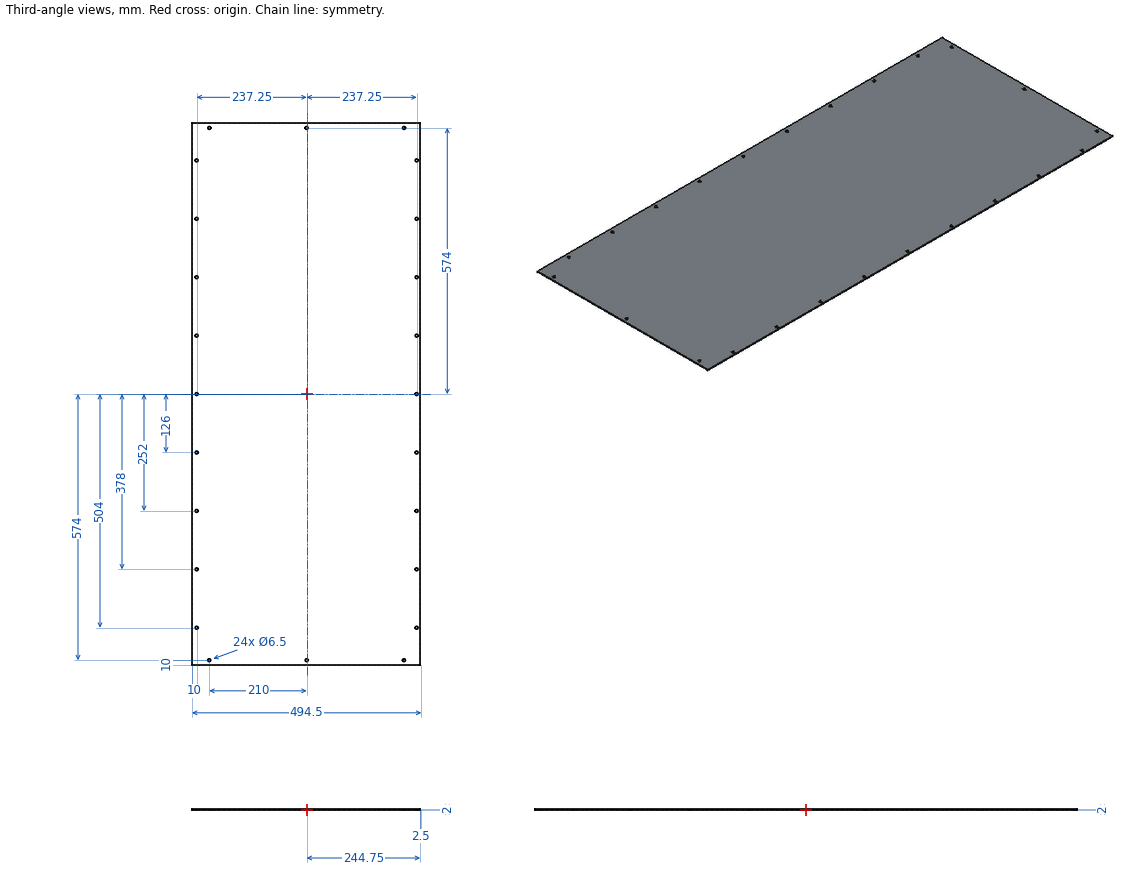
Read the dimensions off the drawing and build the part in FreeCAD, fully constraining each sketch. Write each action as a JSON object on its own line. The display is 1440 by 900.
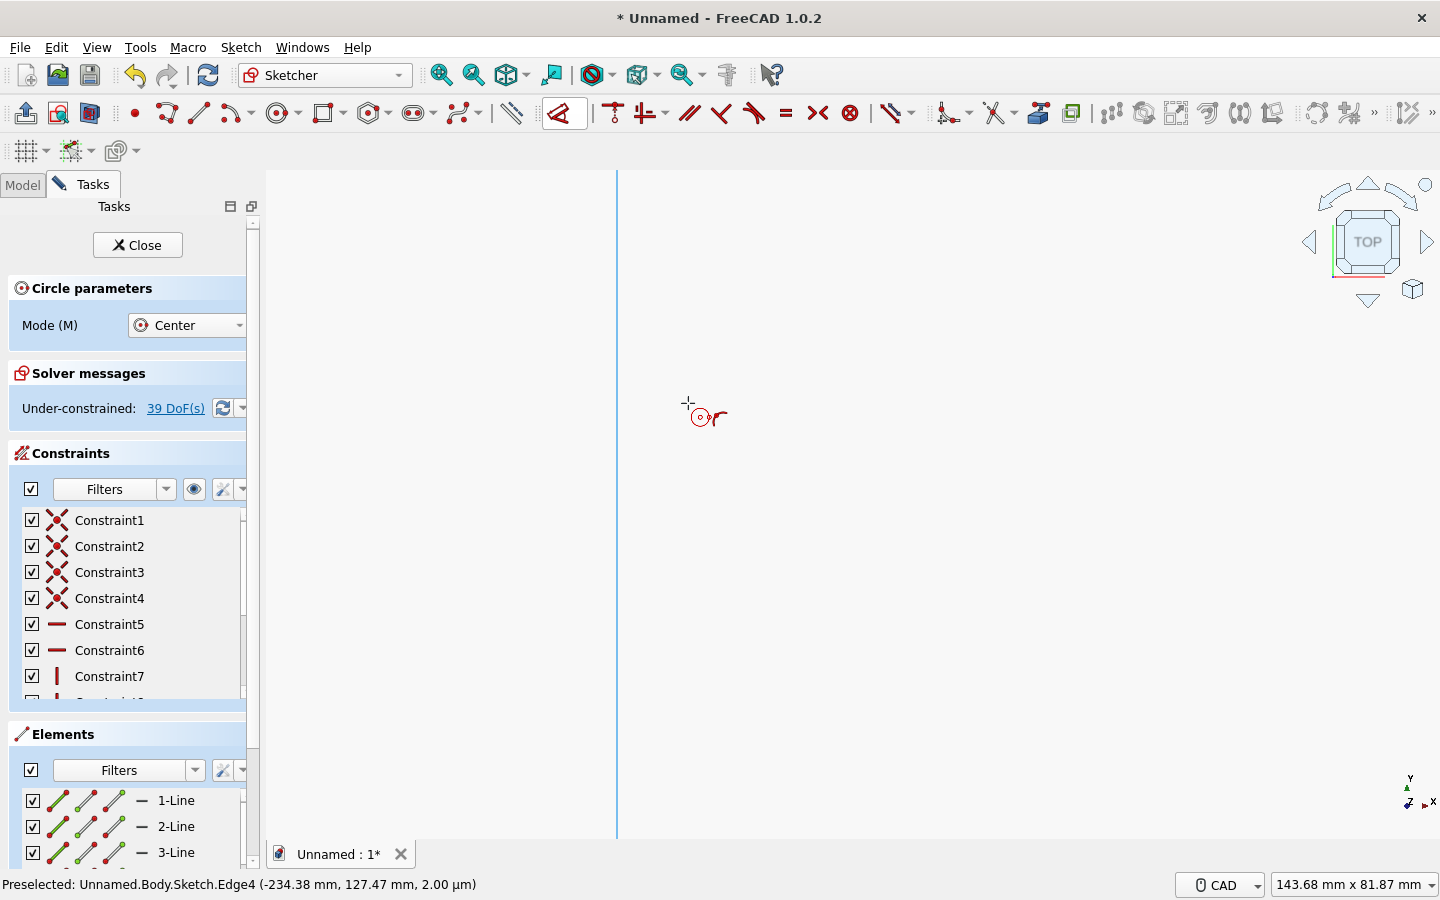
{"action": "scroll", "coordinate": [688, 403], "scroll_direction": "down", "scroll_amount": 15}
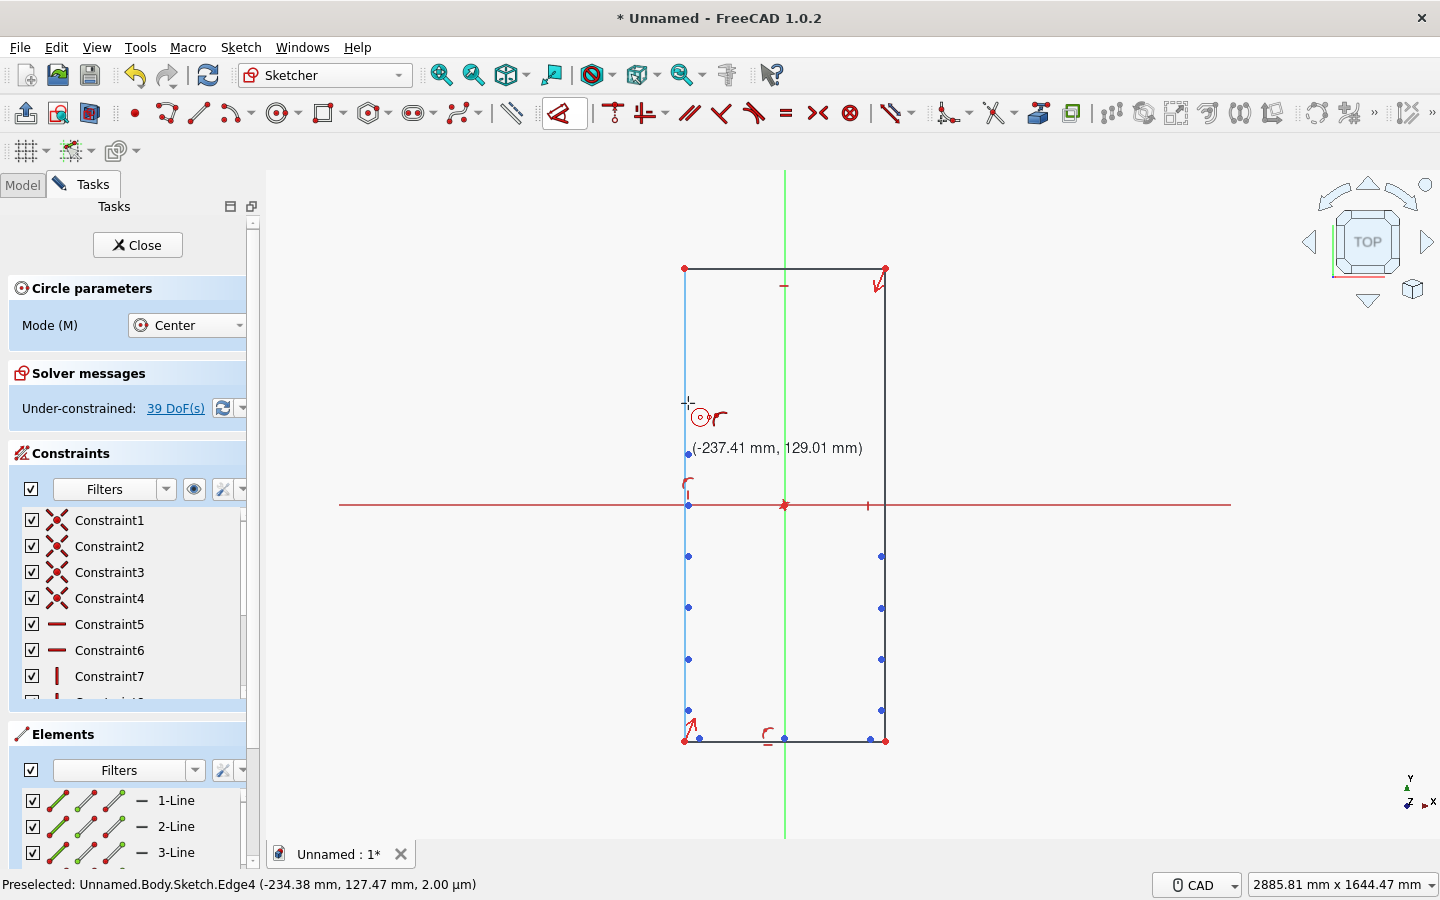
{"action": "scroll", "coordinate": [688, 403], "scroll_direction": "up", "scroll_amount": 7}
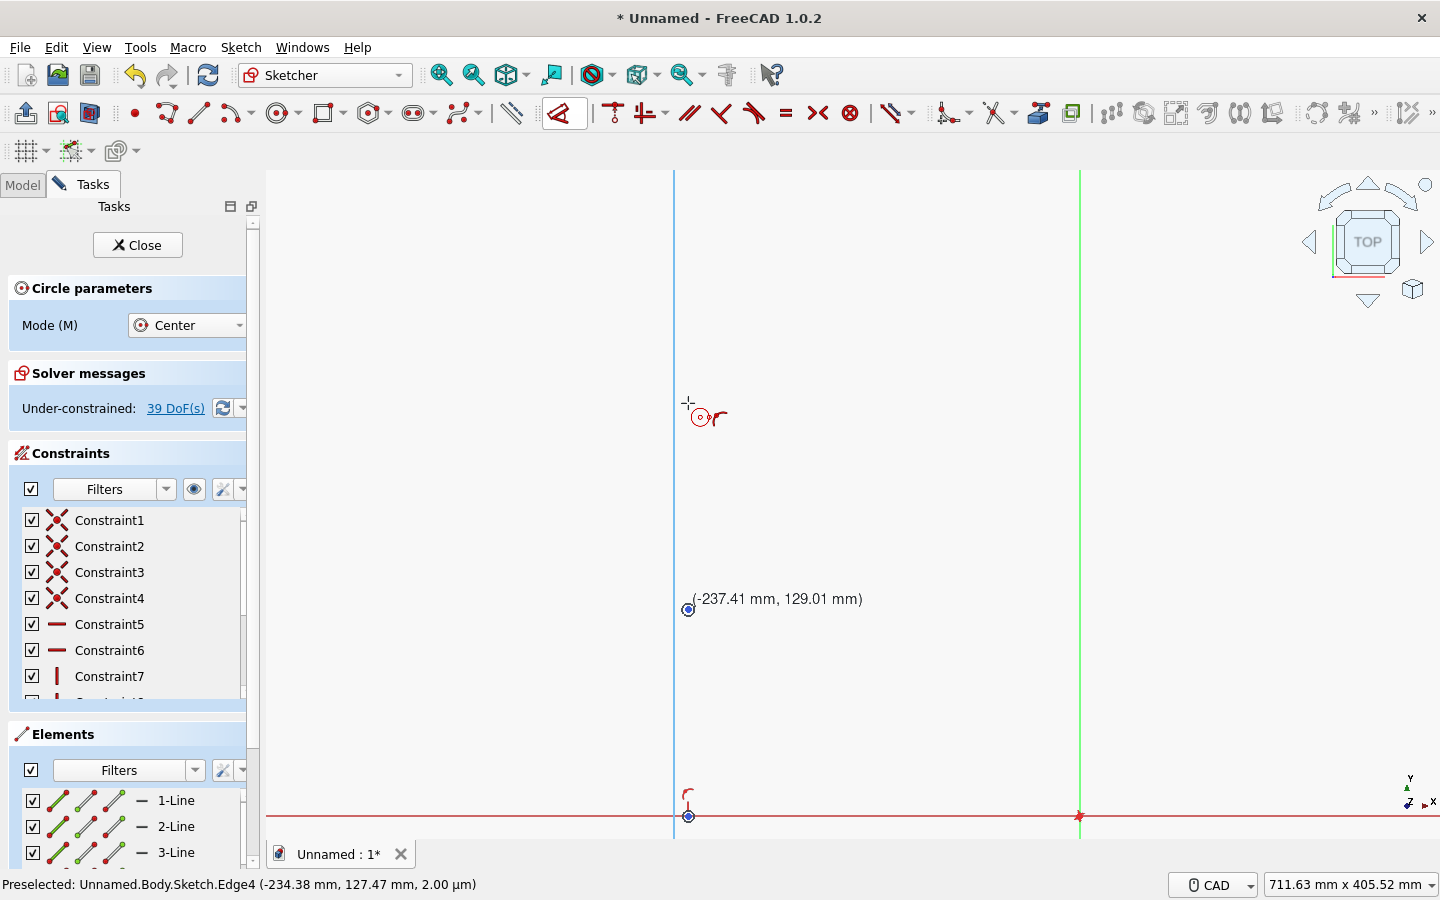
{"action": "left_click", "coordinate": [689, 401]}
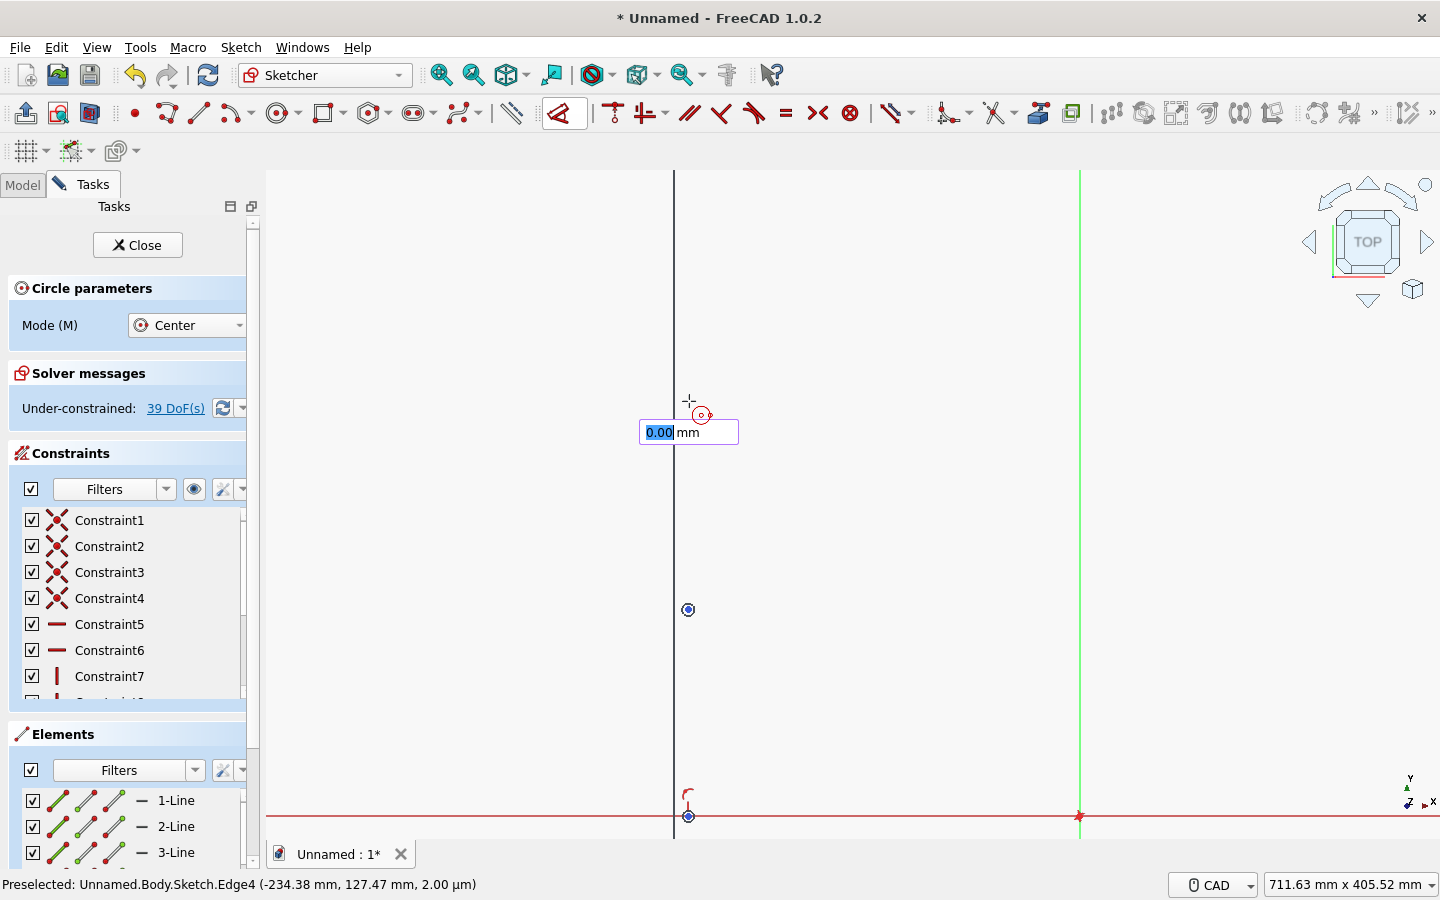
{"action": "scroll", "coordinate": [692, 397], "scroll_direction": "up", "scroll_amount": 6}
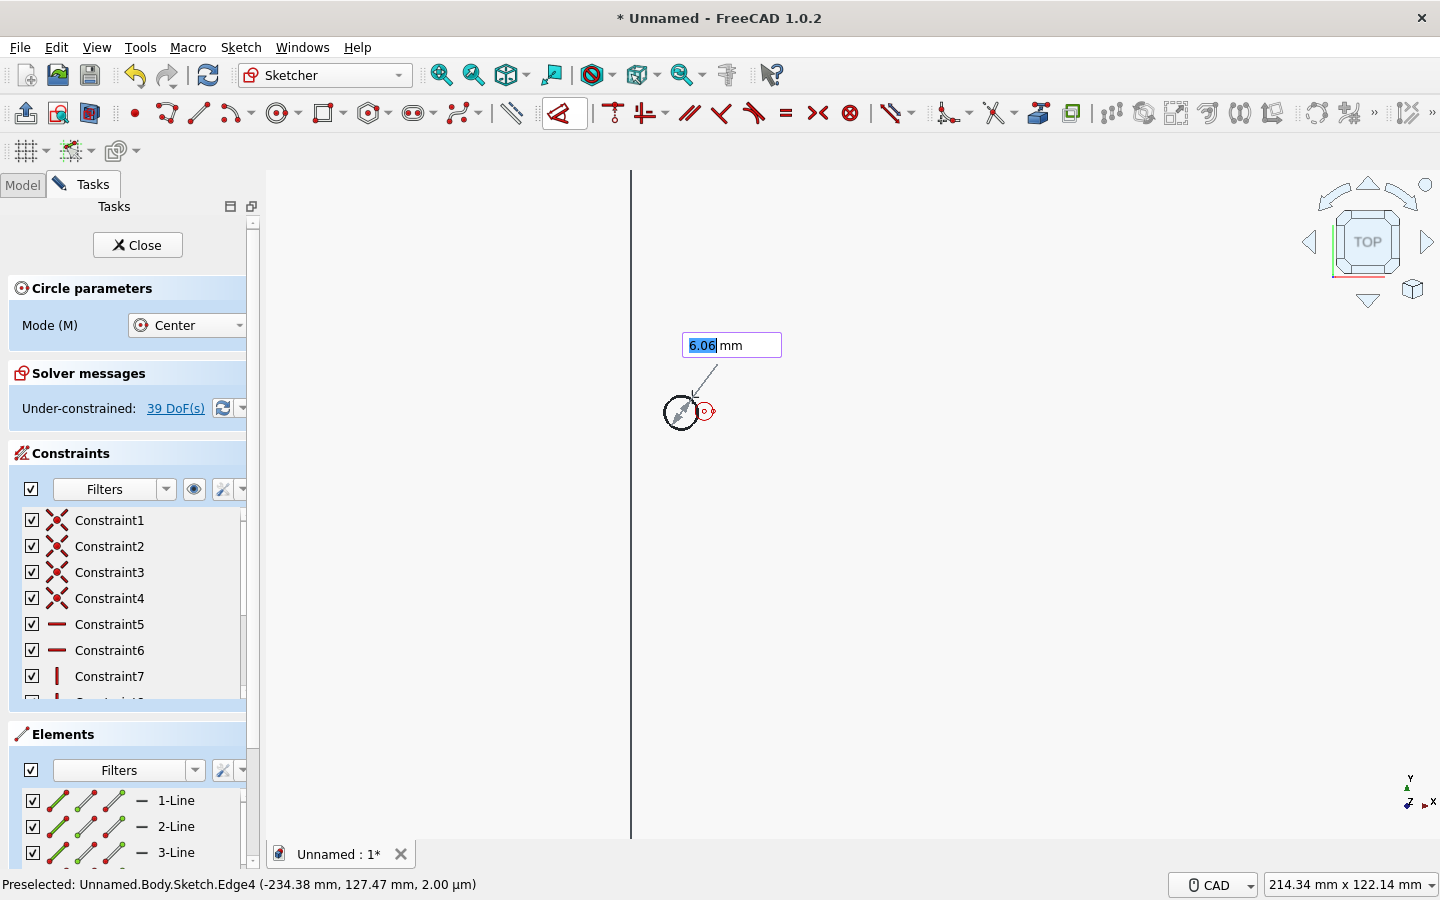
{"action": "left_click", "coordinate": [692, 396]}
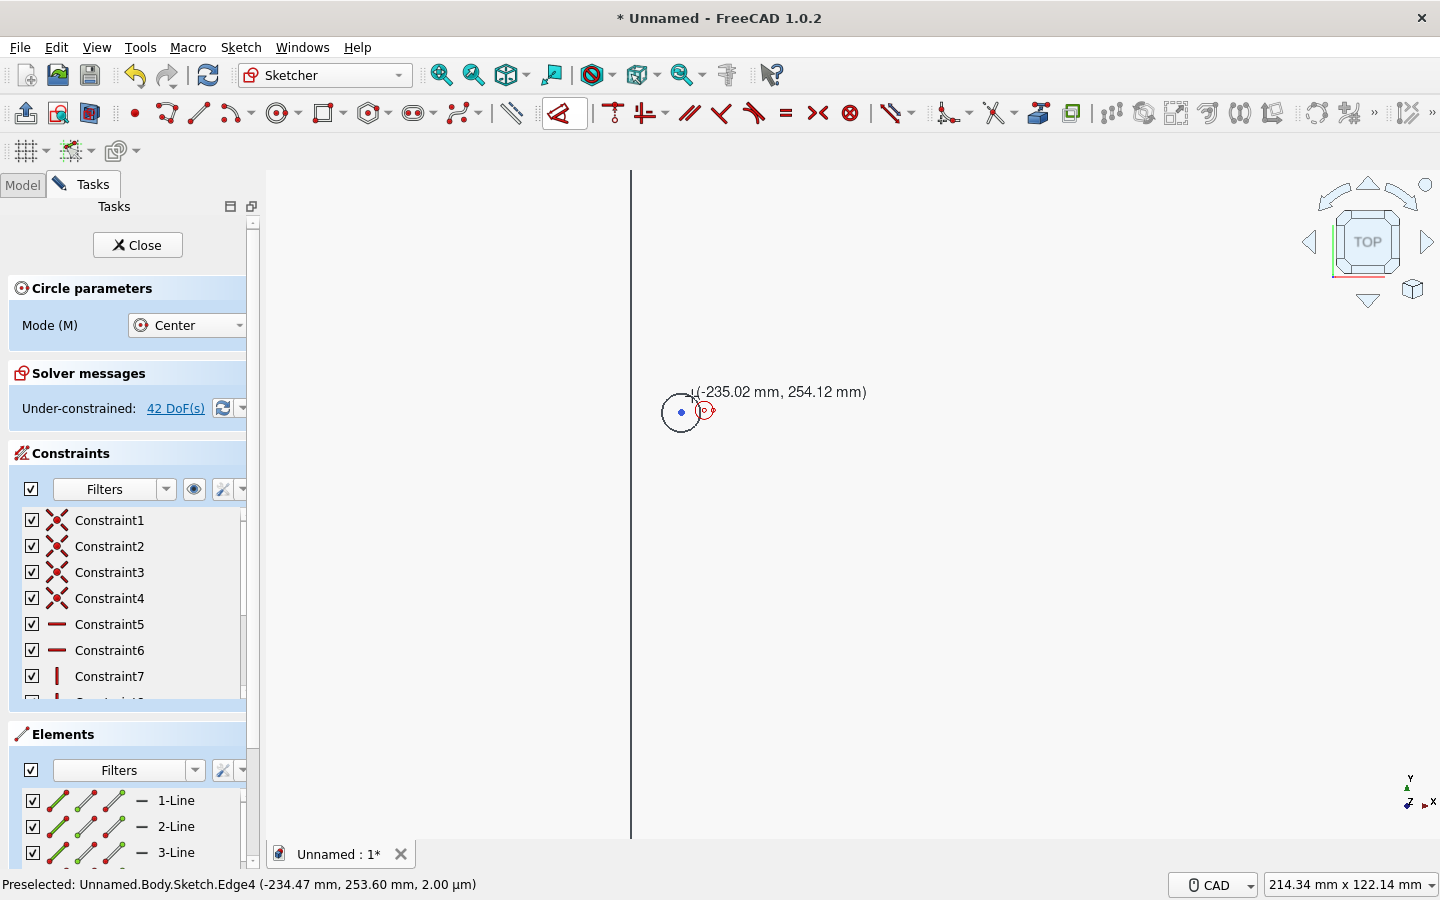
{"action": "scroll", "coordinate": [689, 401], "scroll_direction": "down", "scroll_amount": 13}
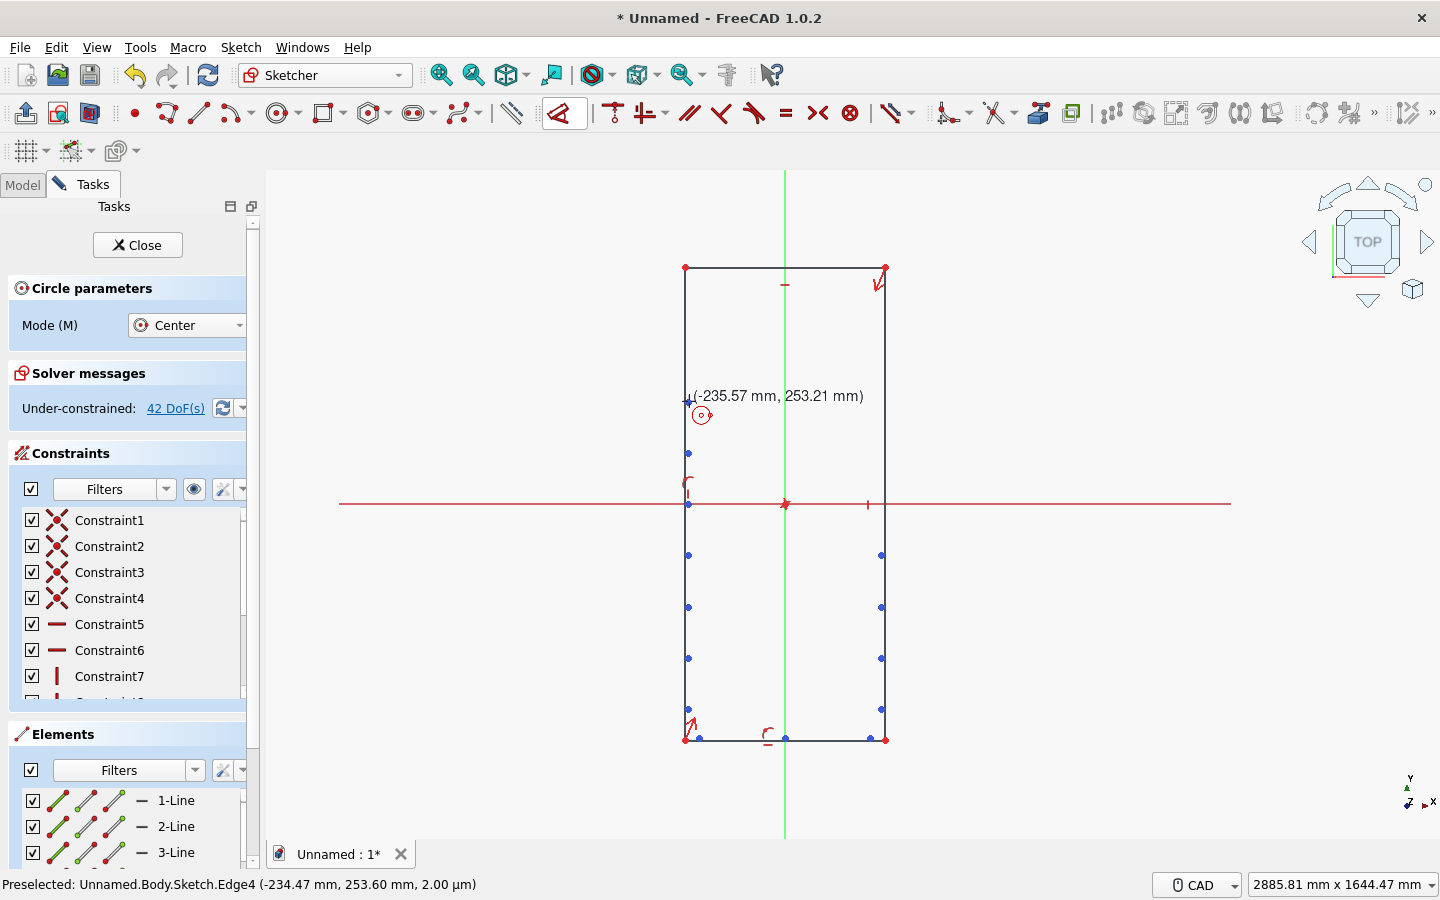
{"action": "scroll", "coordinate": [689, 351], "scroll_direction": "up", "scroll_amount": 15}